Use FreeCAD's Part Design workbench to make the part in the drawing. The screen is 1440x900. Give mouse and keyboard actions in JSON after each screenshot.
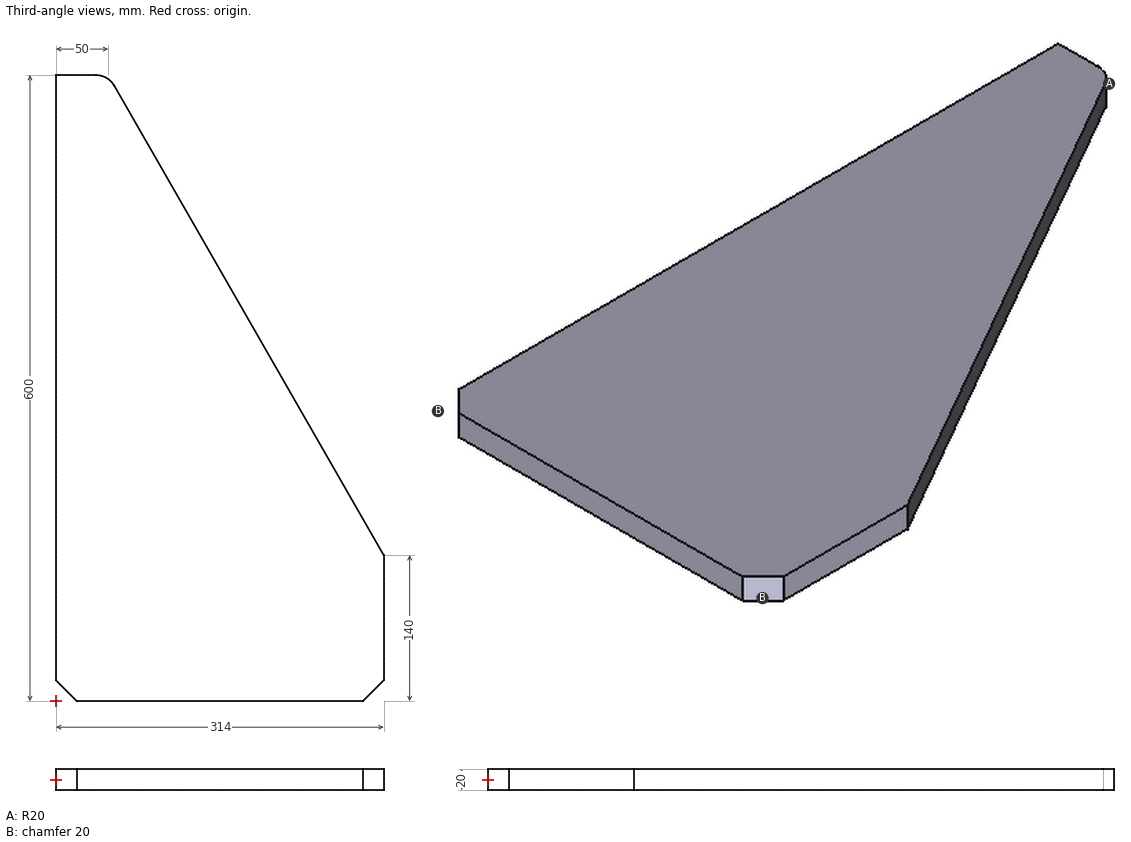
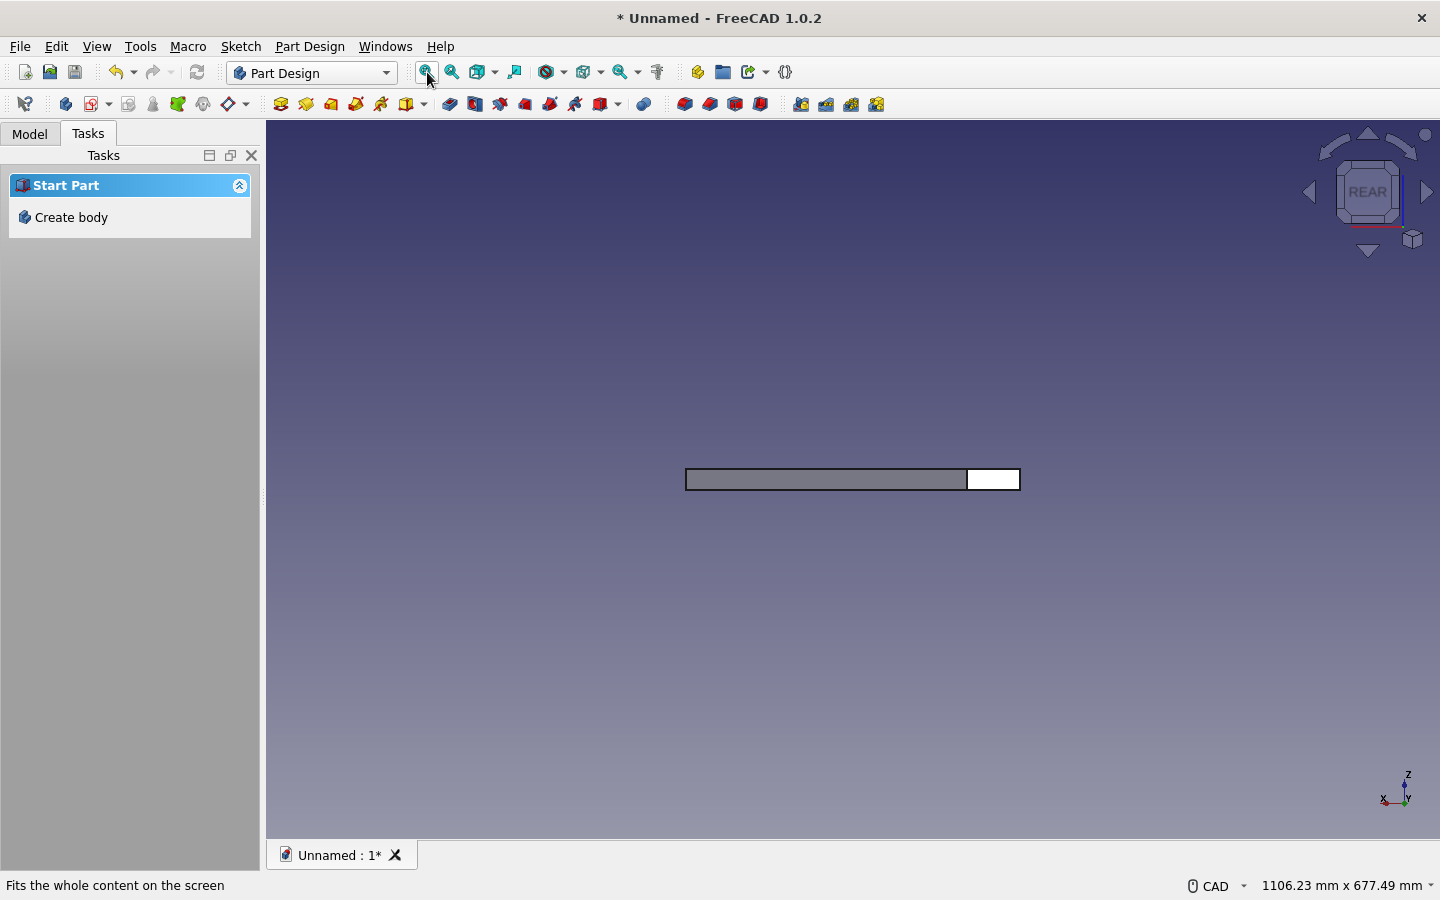
{"action": "left_click", "coordinate": [967, 479]}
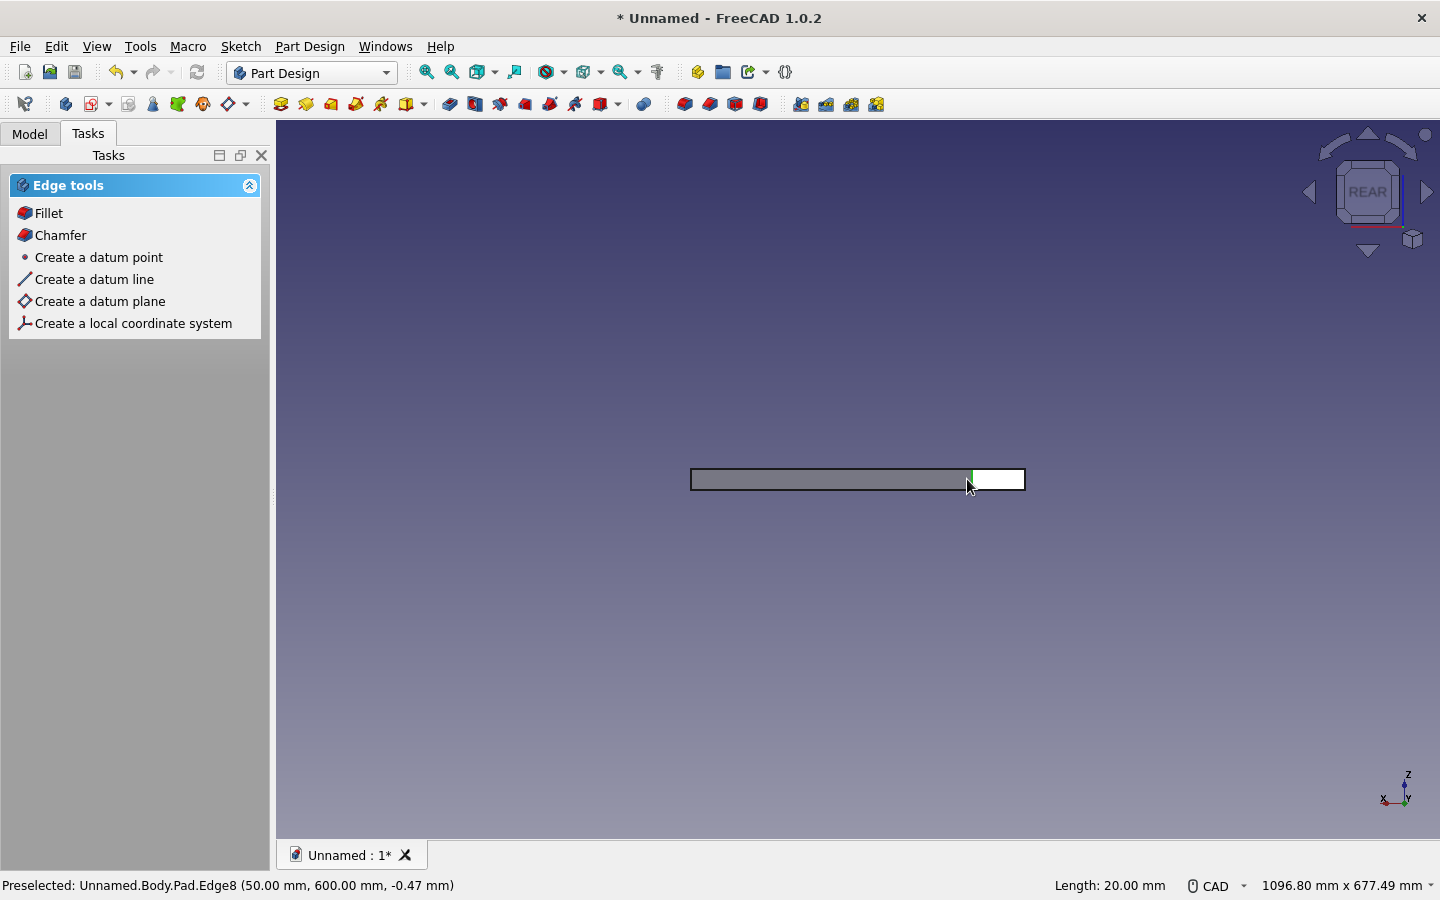
{"action": "left_click", "coordinate": [685, 104]}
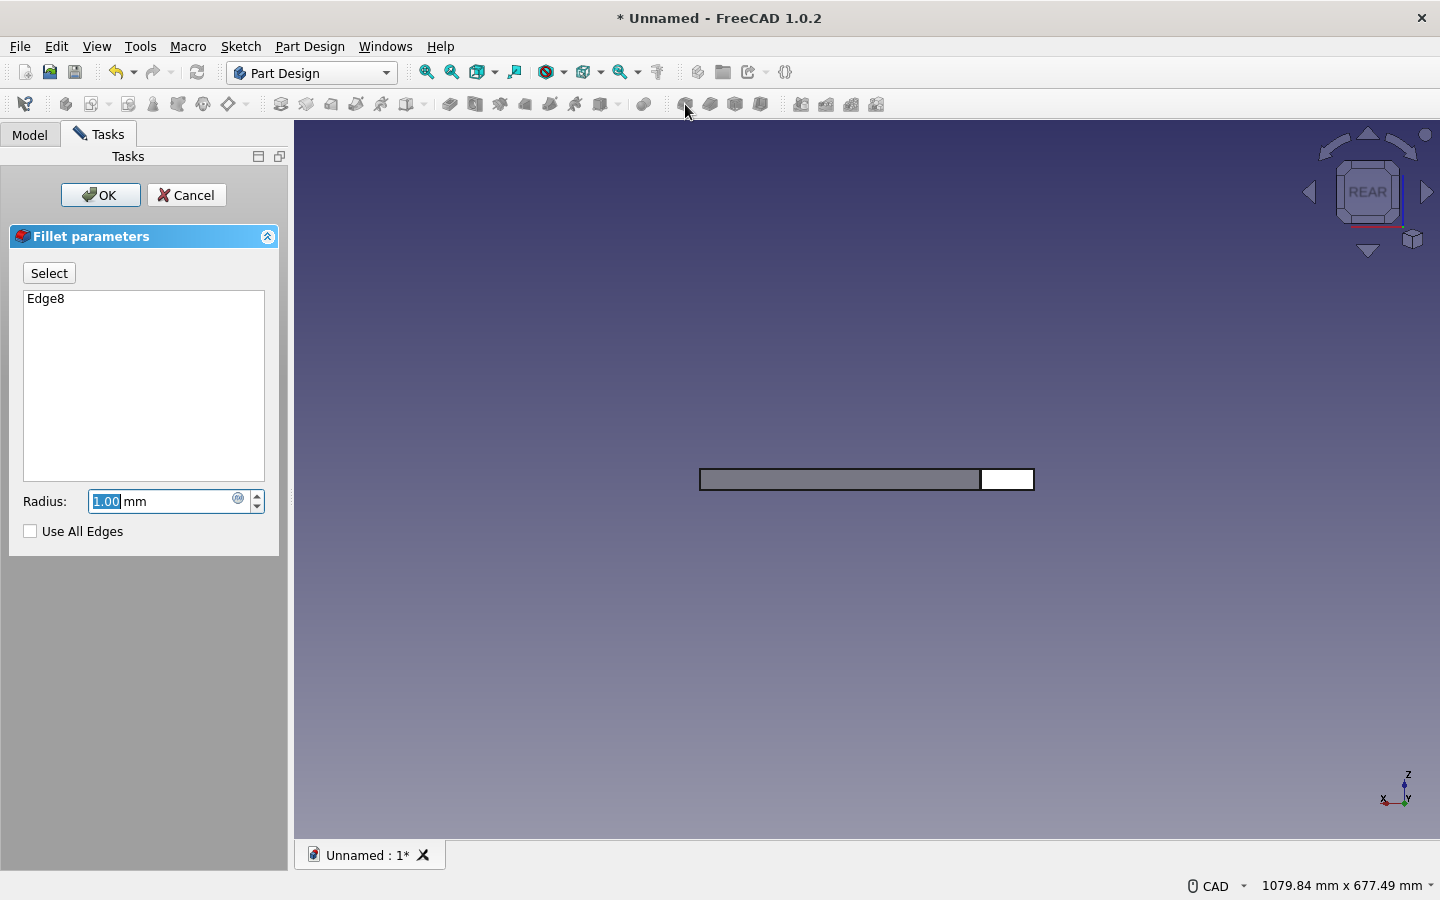
{"action": "type", "text": "20"}
{"action": "key", "text": "Tab"}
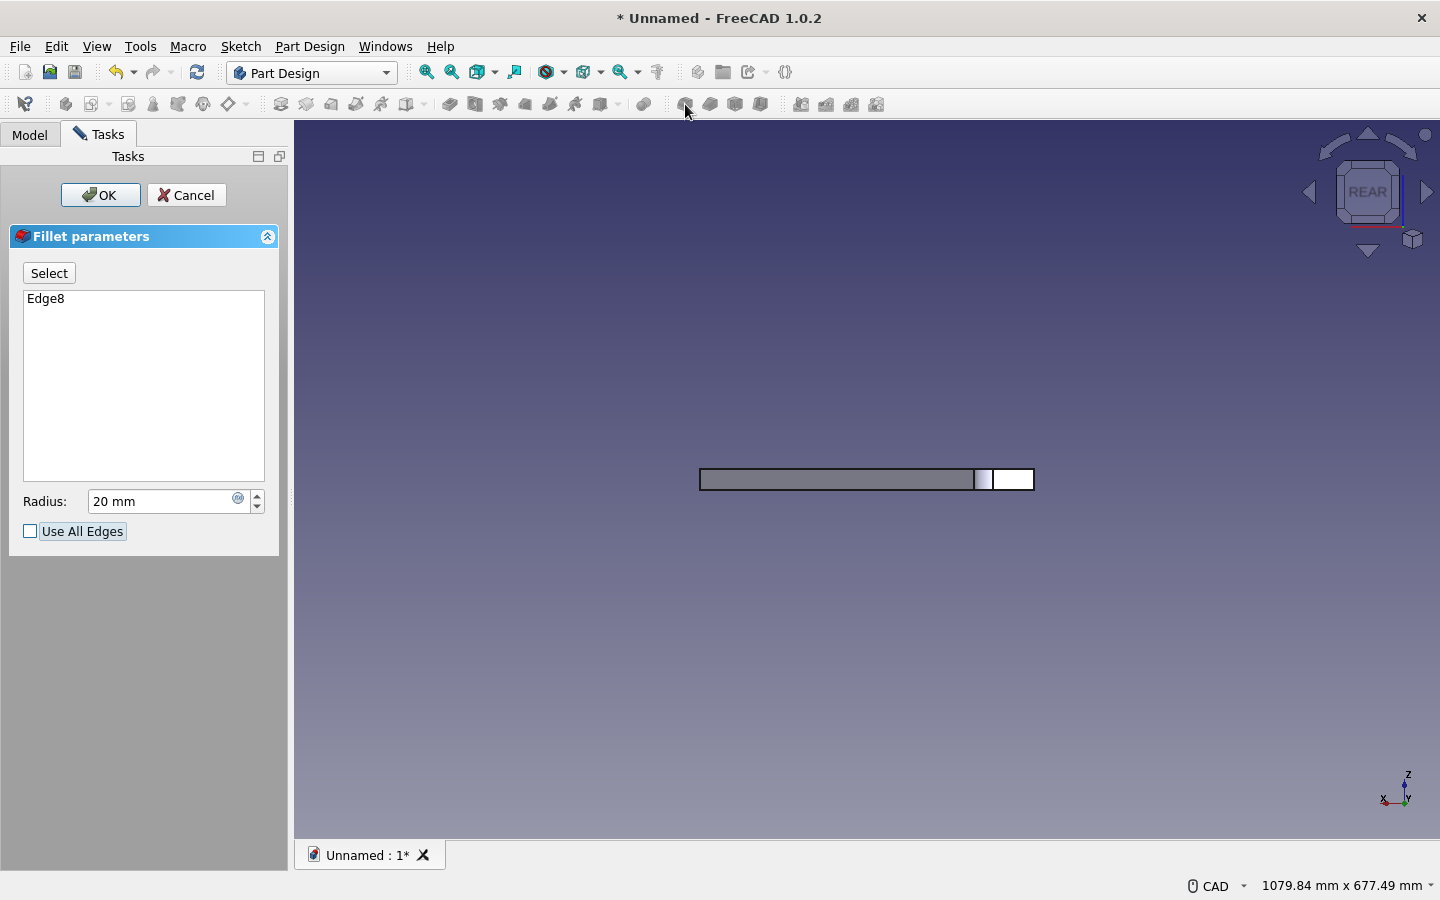
{"action": "left_click", "coordinate": [101, 195]}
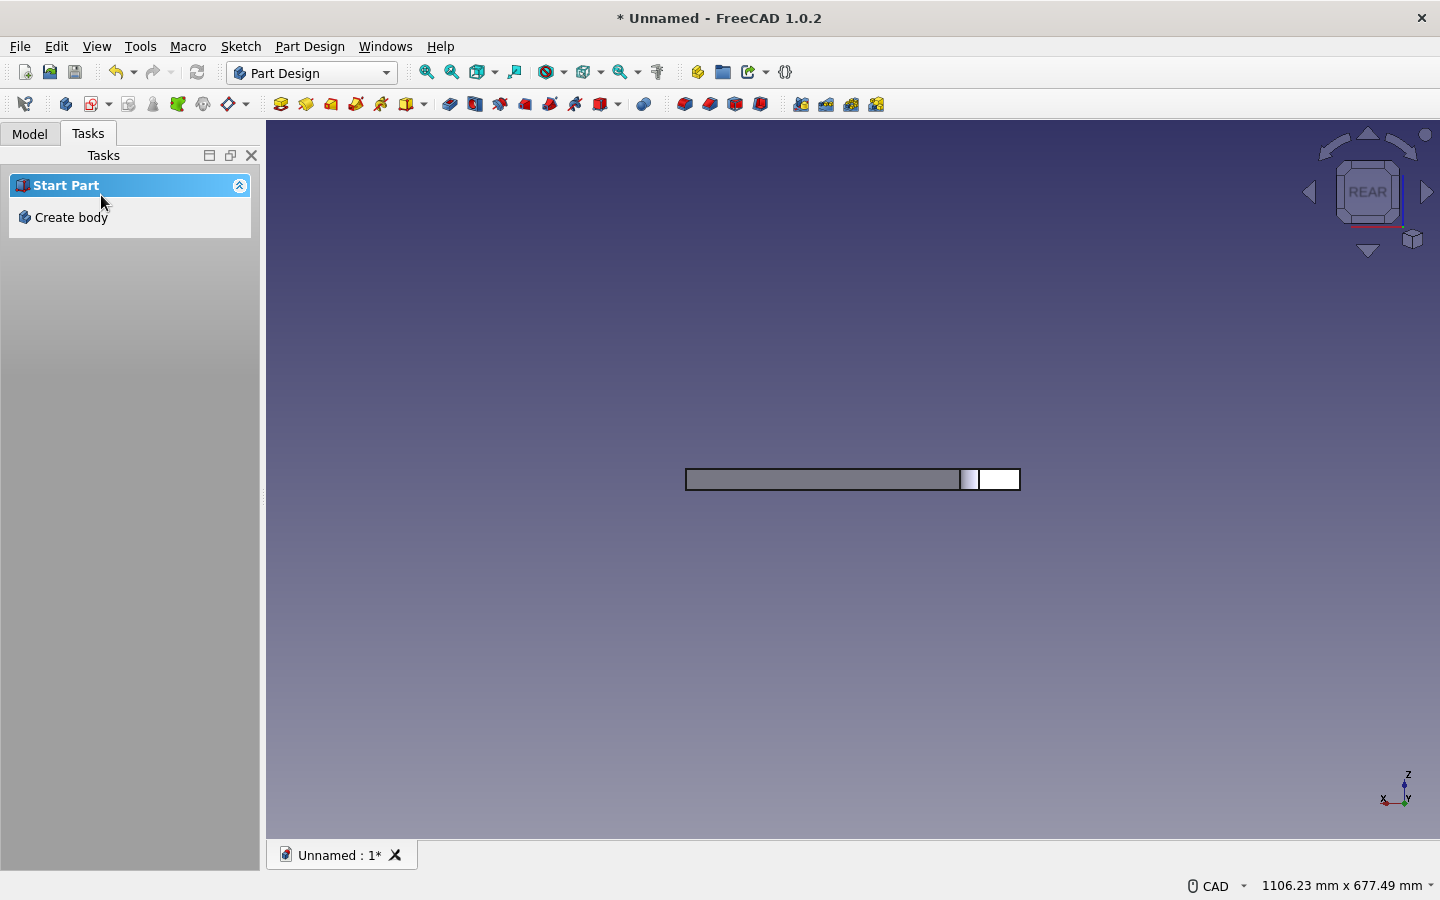
{"action": "left_click", "coordinate": [427, 72]}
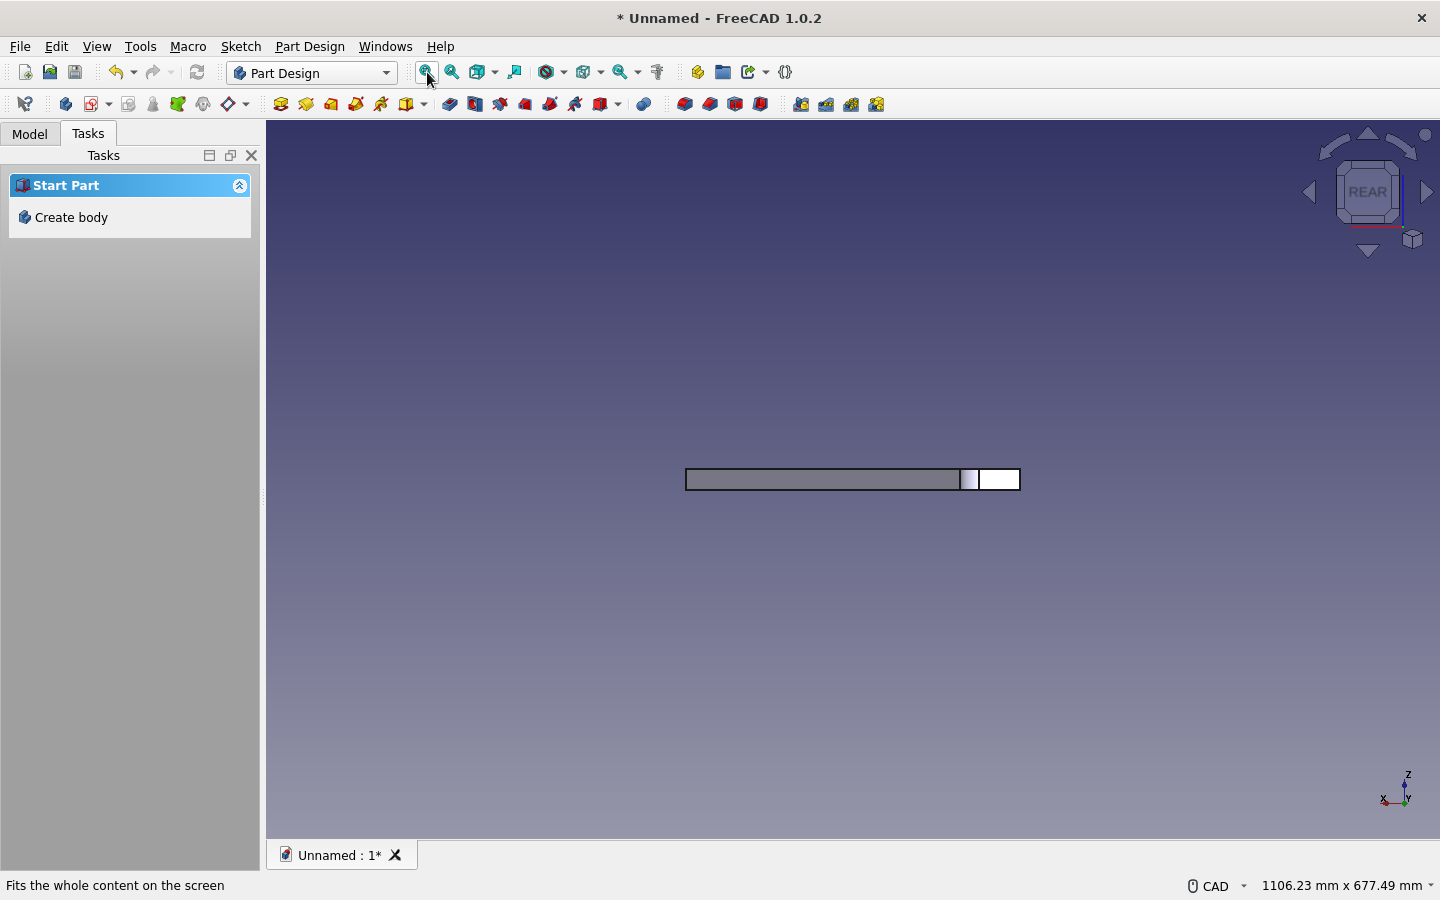
{"action": "scroll", "coordinate": [686, 479], "scroll_direction": "up", "scroll_amount": 4}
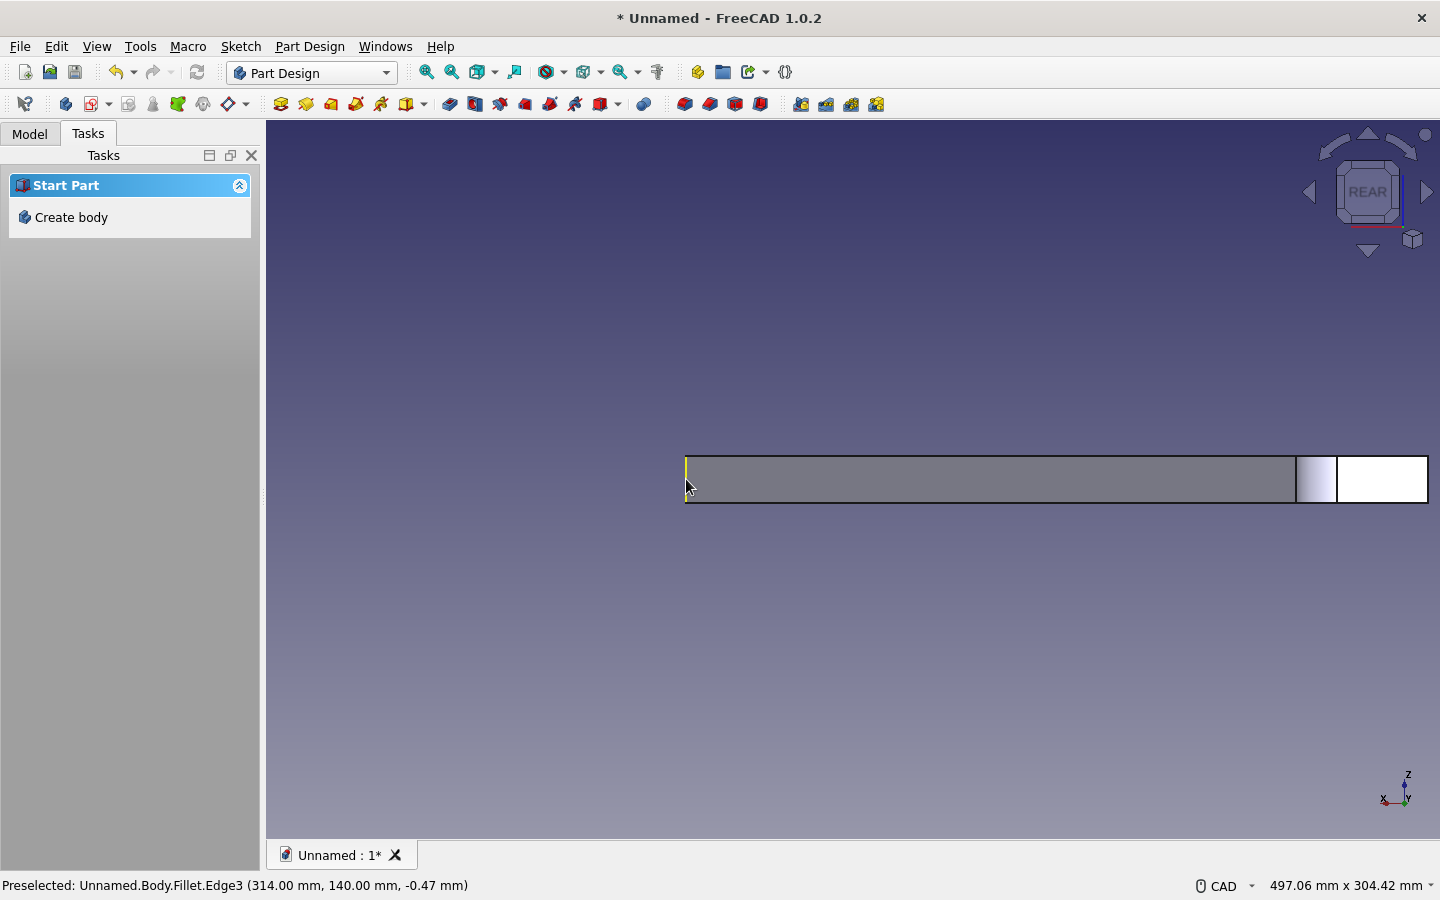
{"action": "key", "text": "v f"}